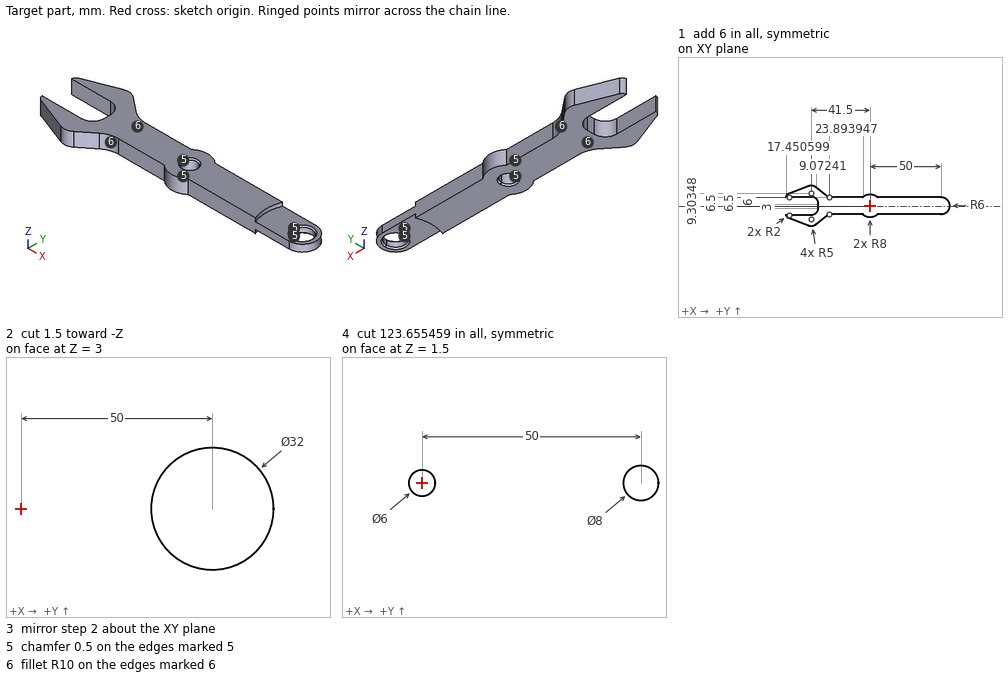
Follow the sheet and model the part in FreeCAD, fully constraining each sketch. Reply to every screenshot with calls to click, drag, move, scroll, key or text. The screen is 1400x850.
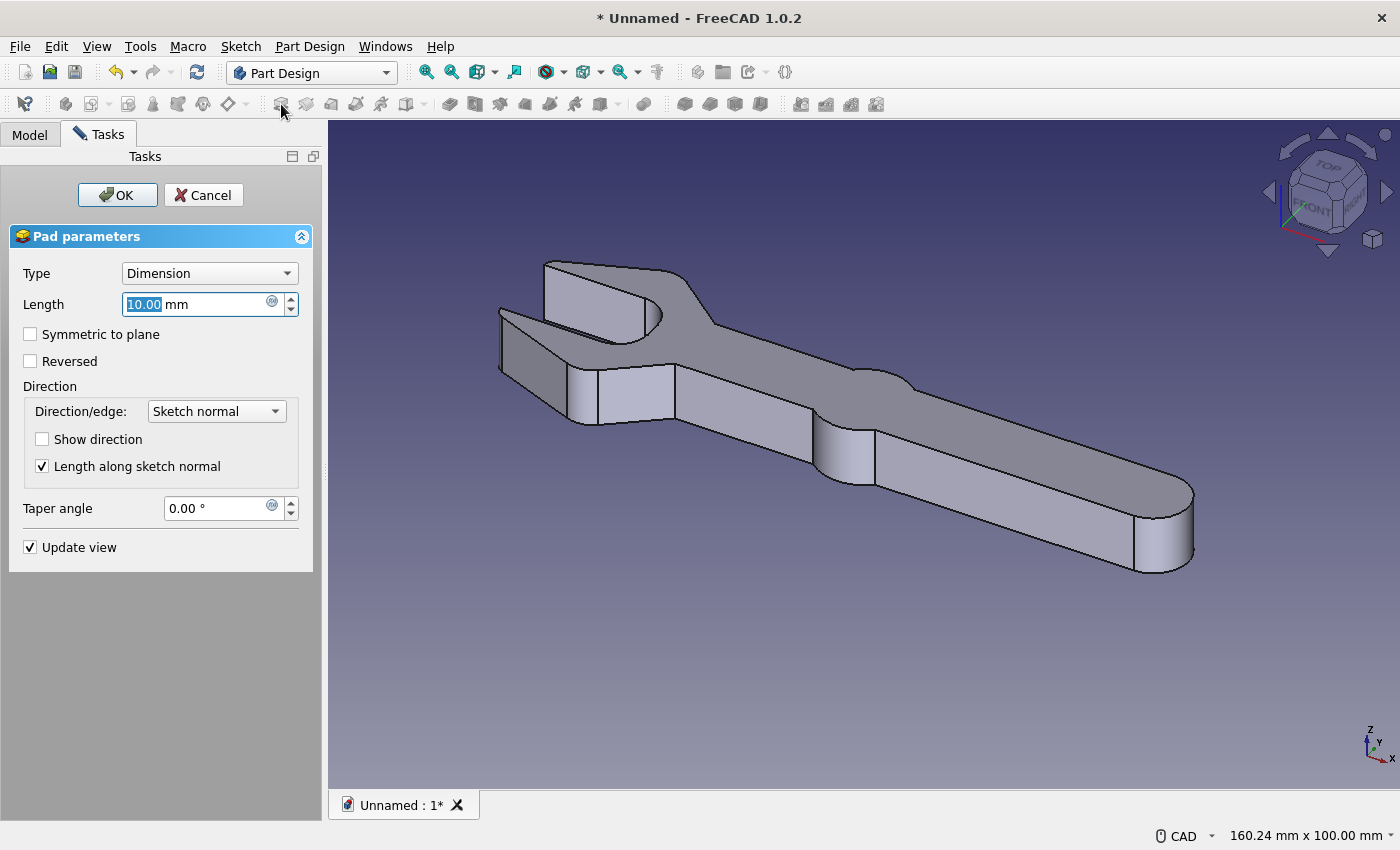
text(6)
key(Tab)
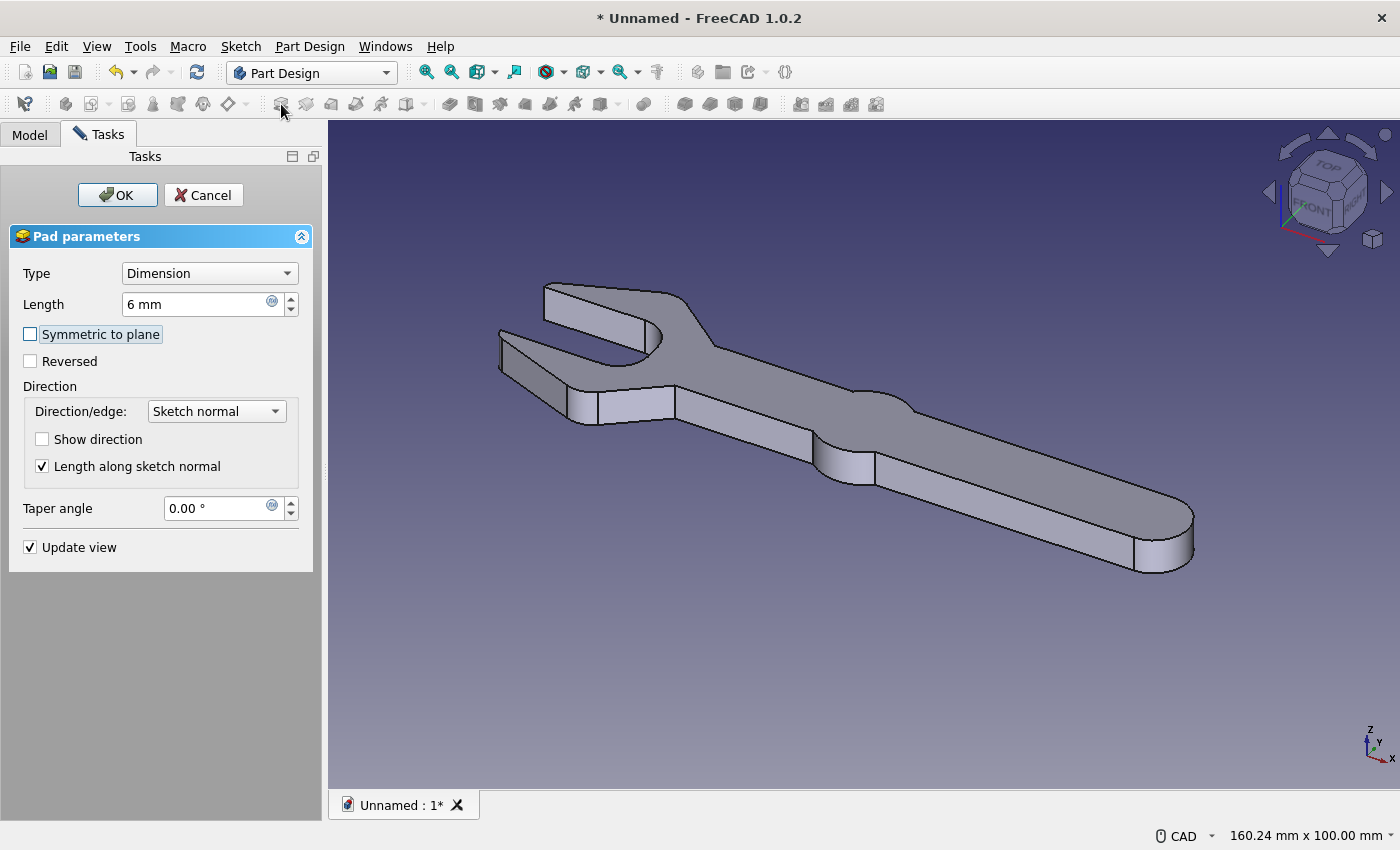
click(31, 334)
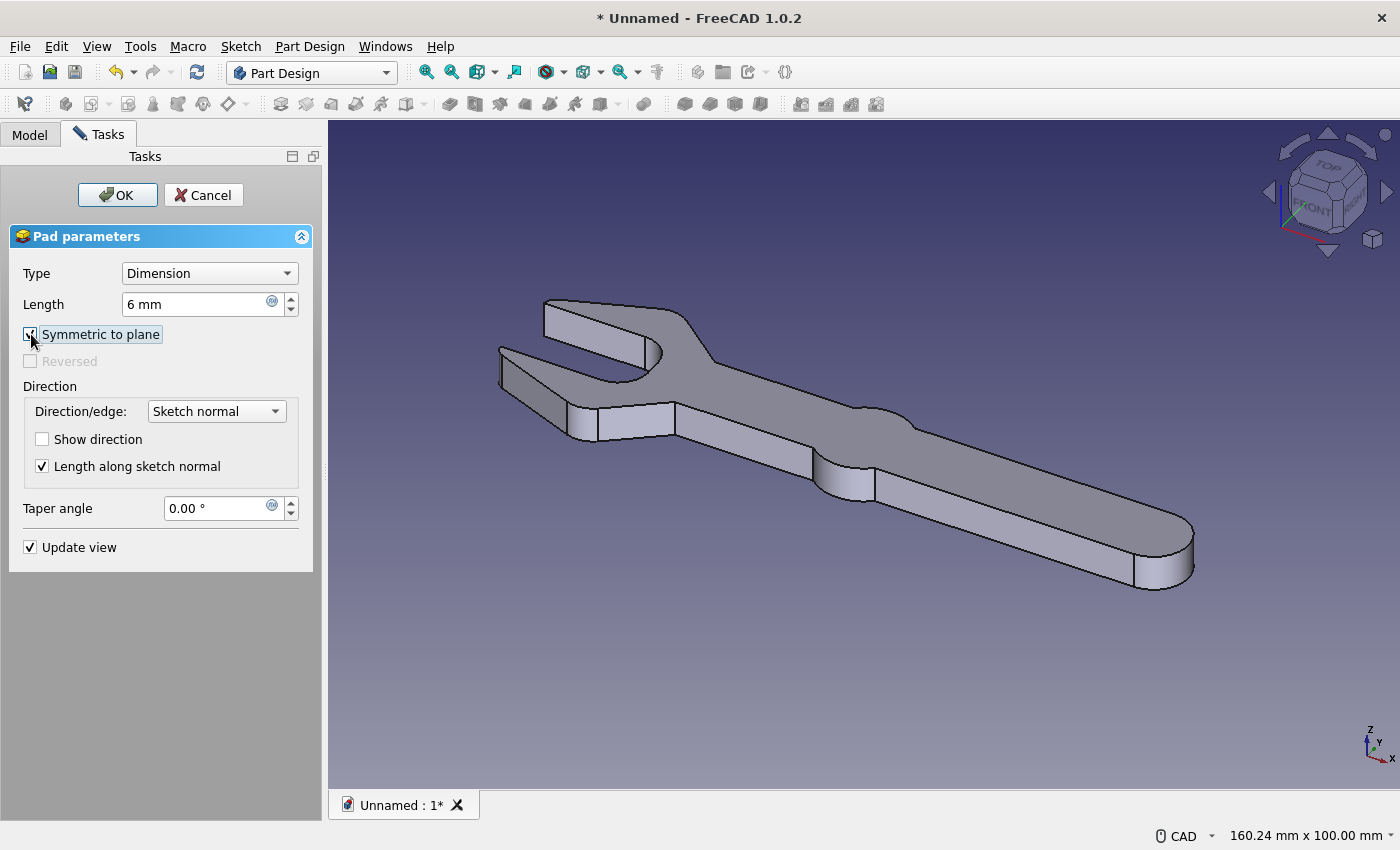
click(118, 195)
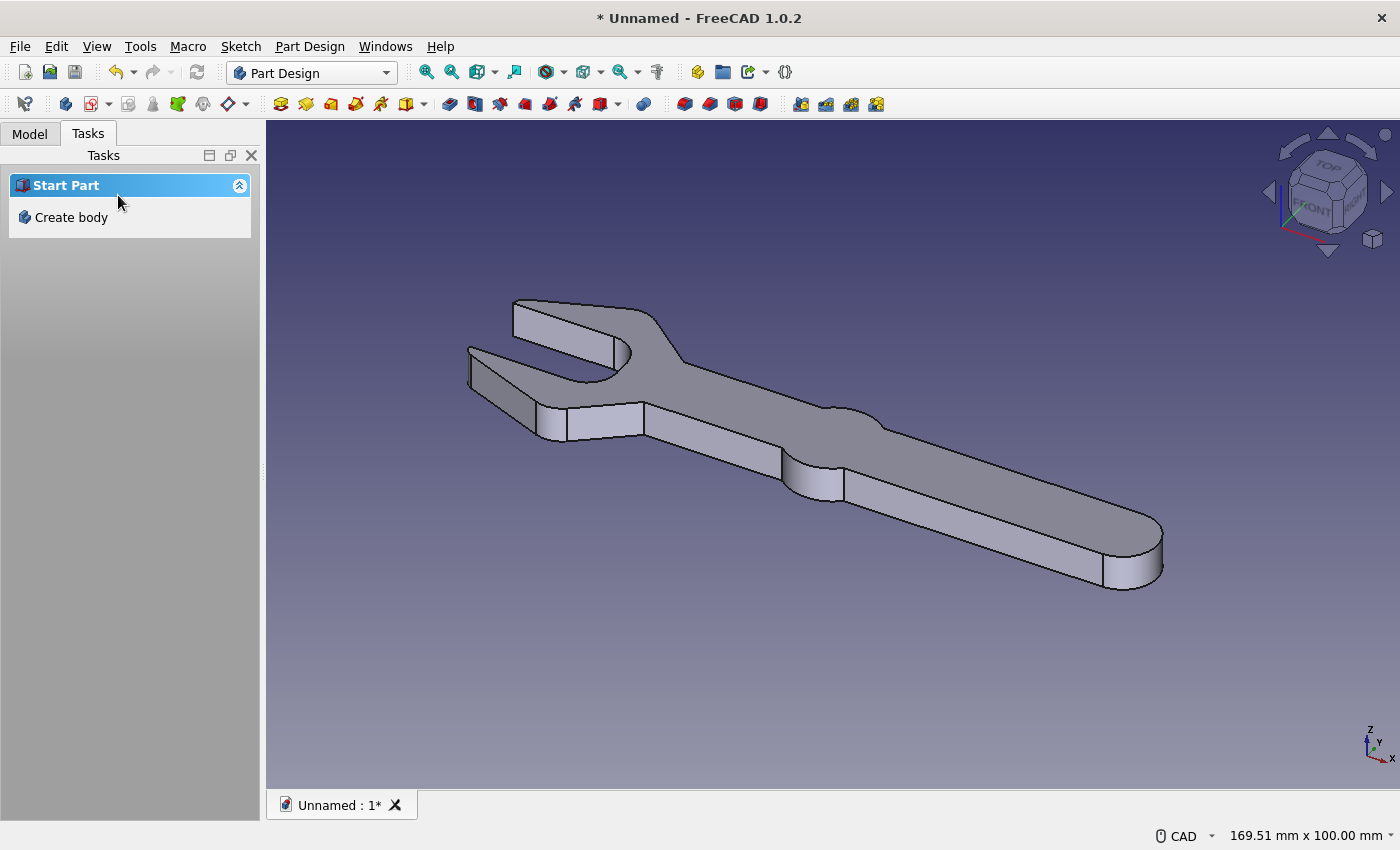
click(824, 434)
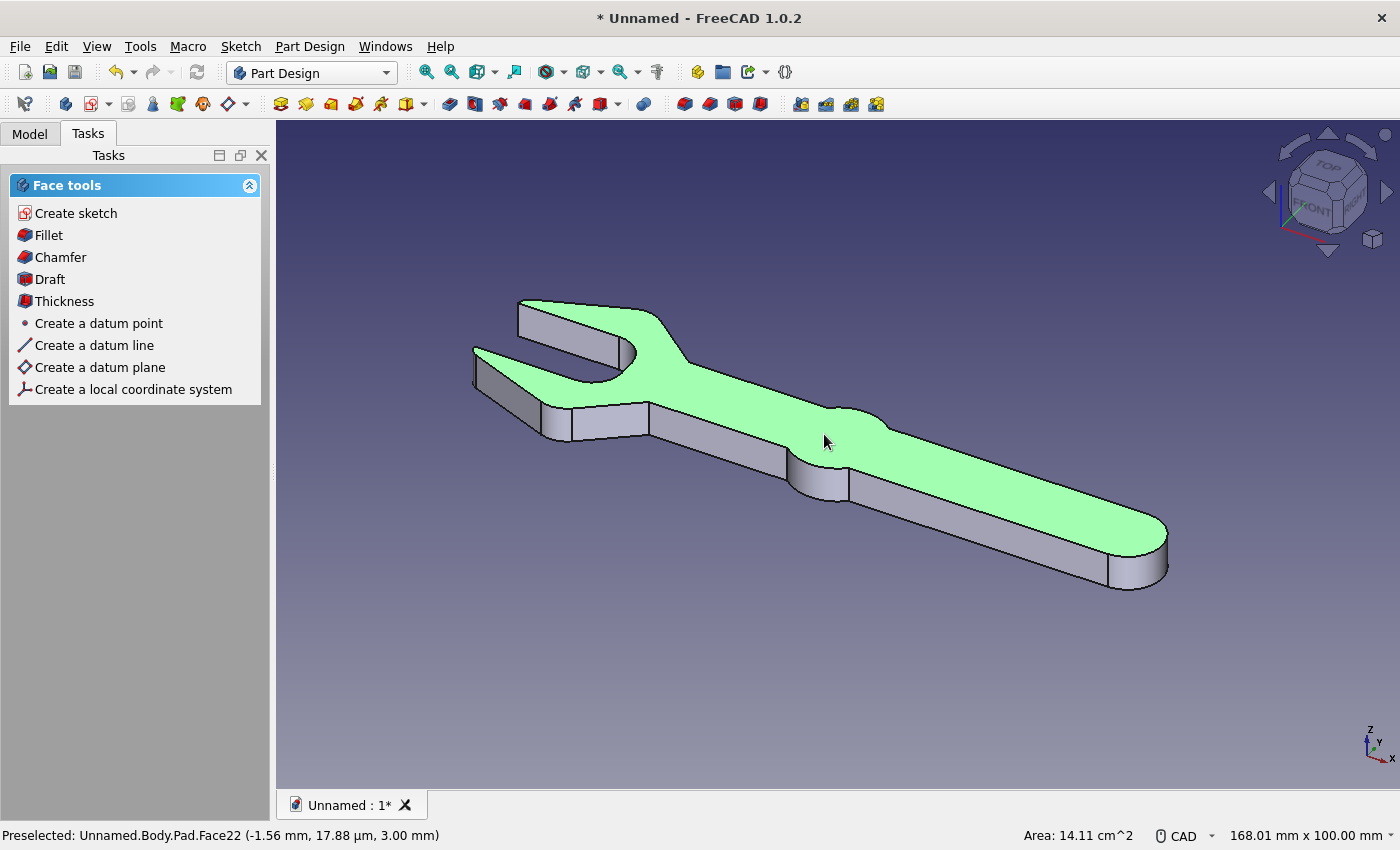
click(90, 104)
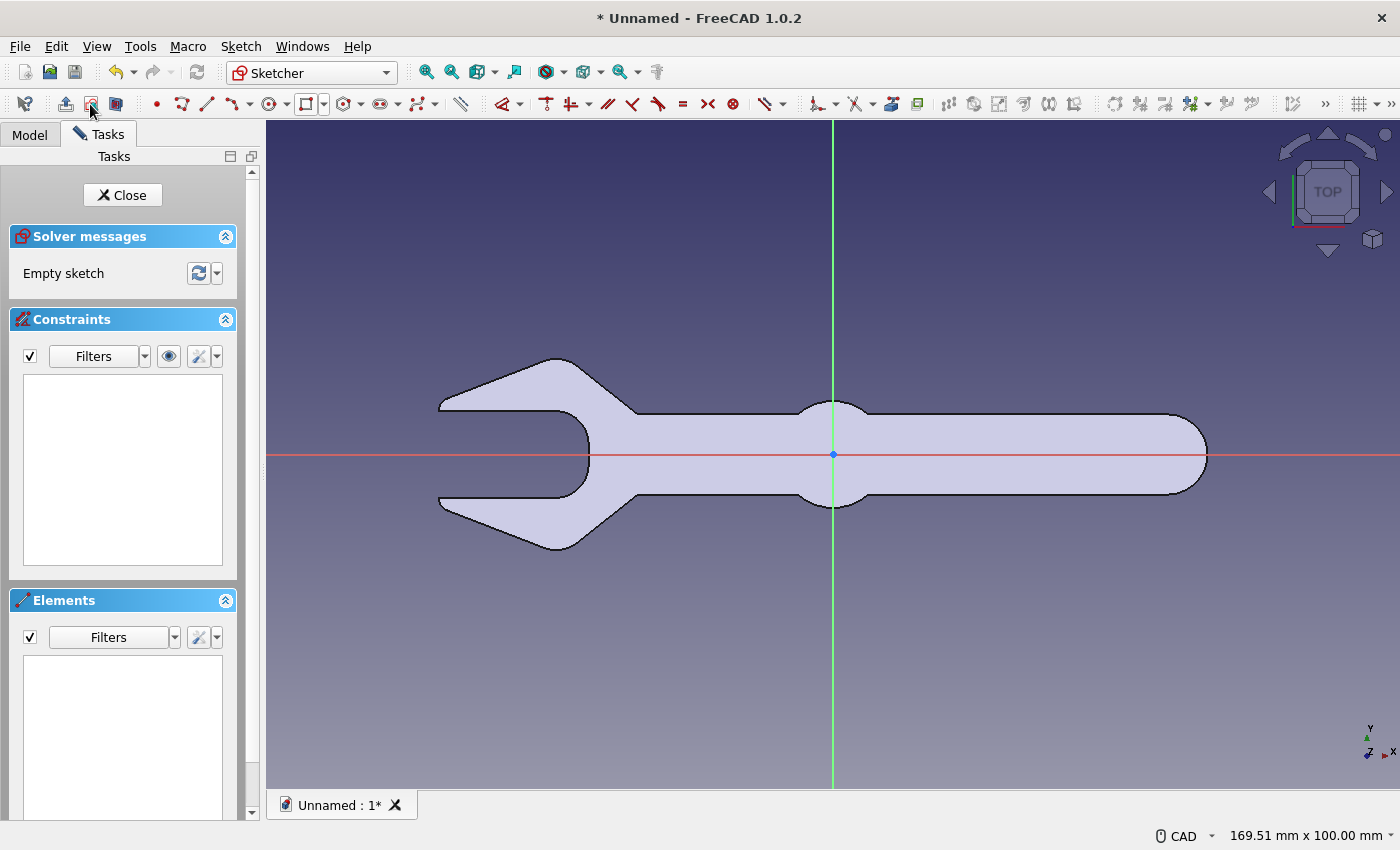
scroll(294, 455, down, 1)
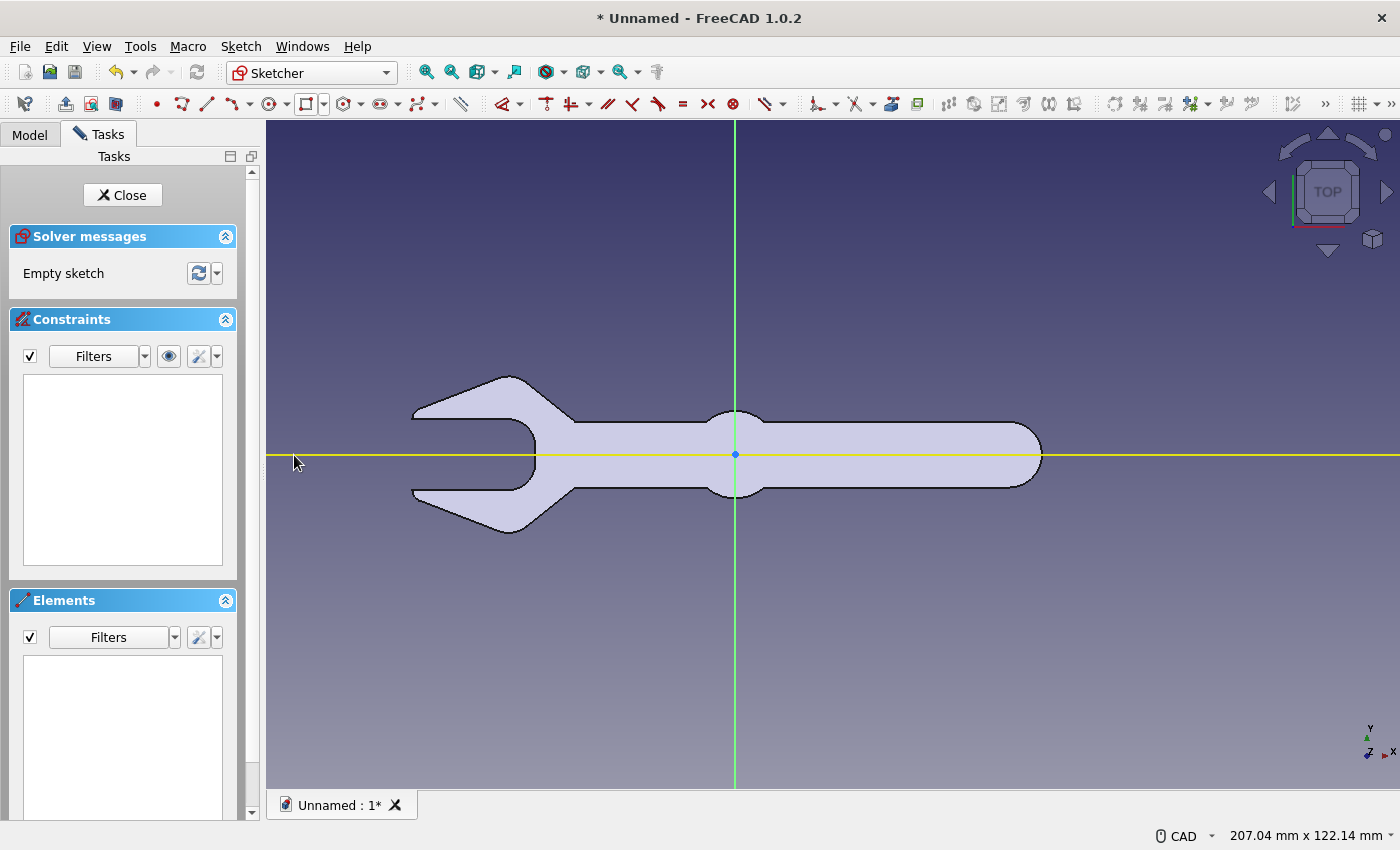
scroll(1100, 455, up, 3)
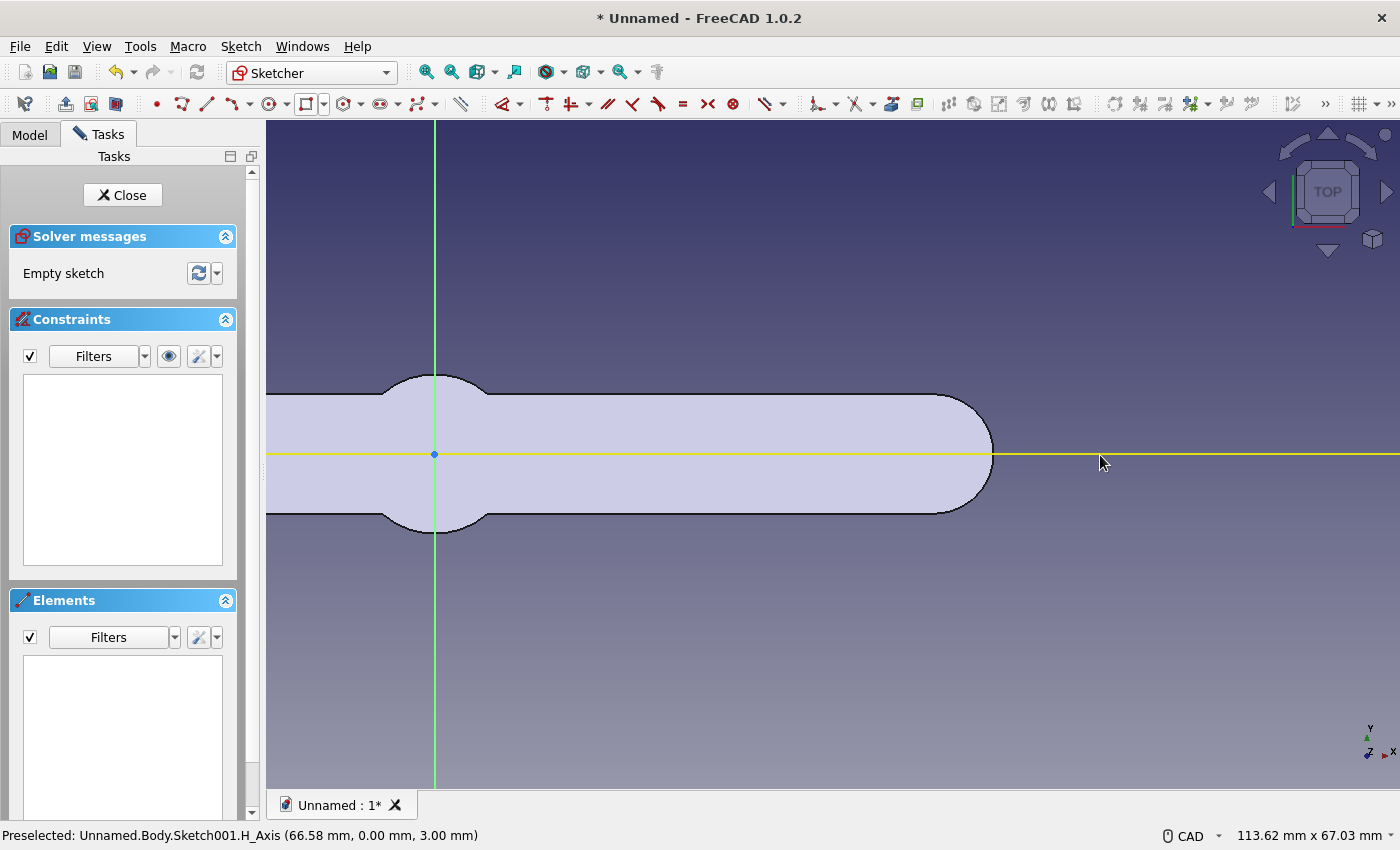
click(268, 104)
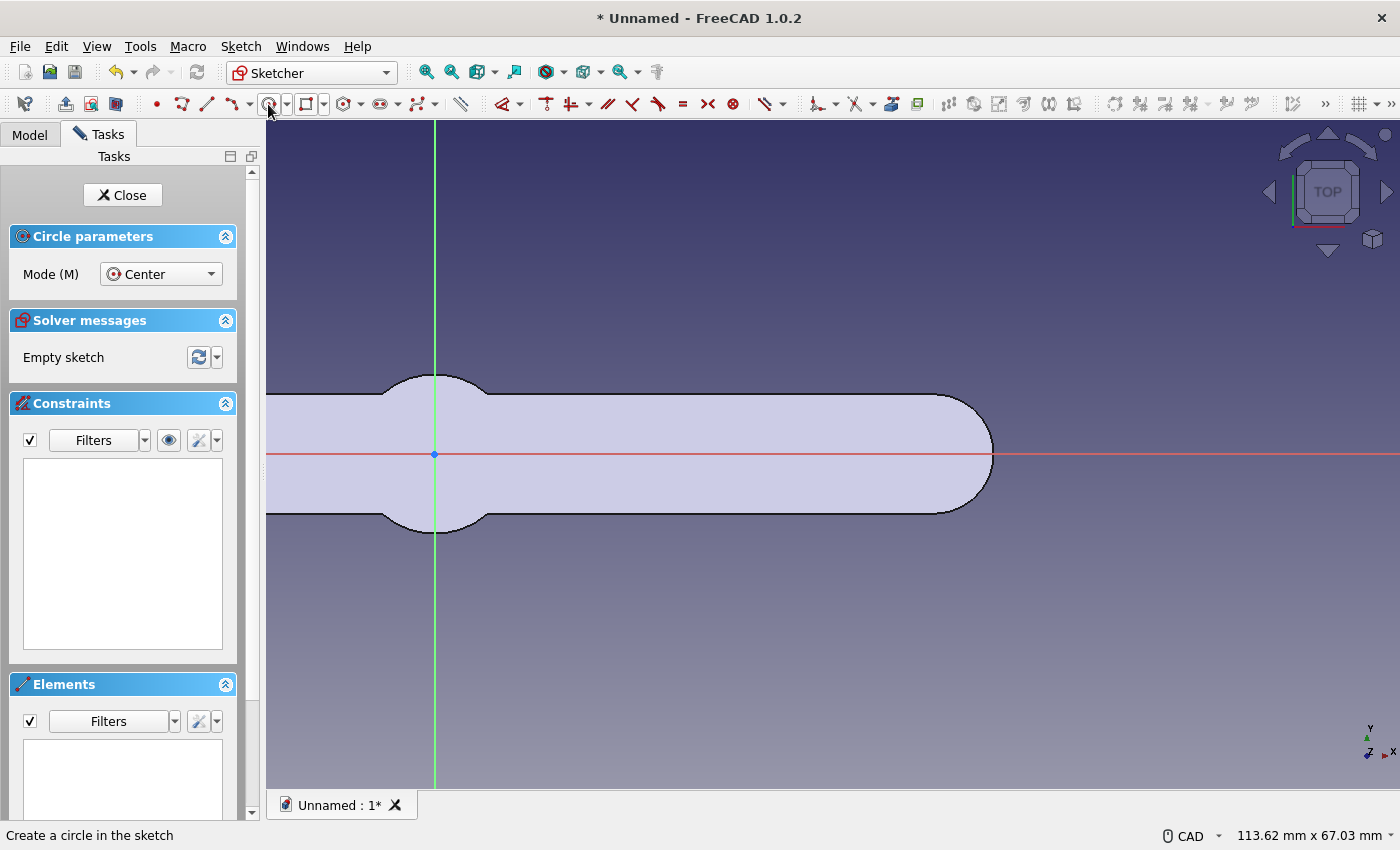
click(934, 454)
move(1047, 341)